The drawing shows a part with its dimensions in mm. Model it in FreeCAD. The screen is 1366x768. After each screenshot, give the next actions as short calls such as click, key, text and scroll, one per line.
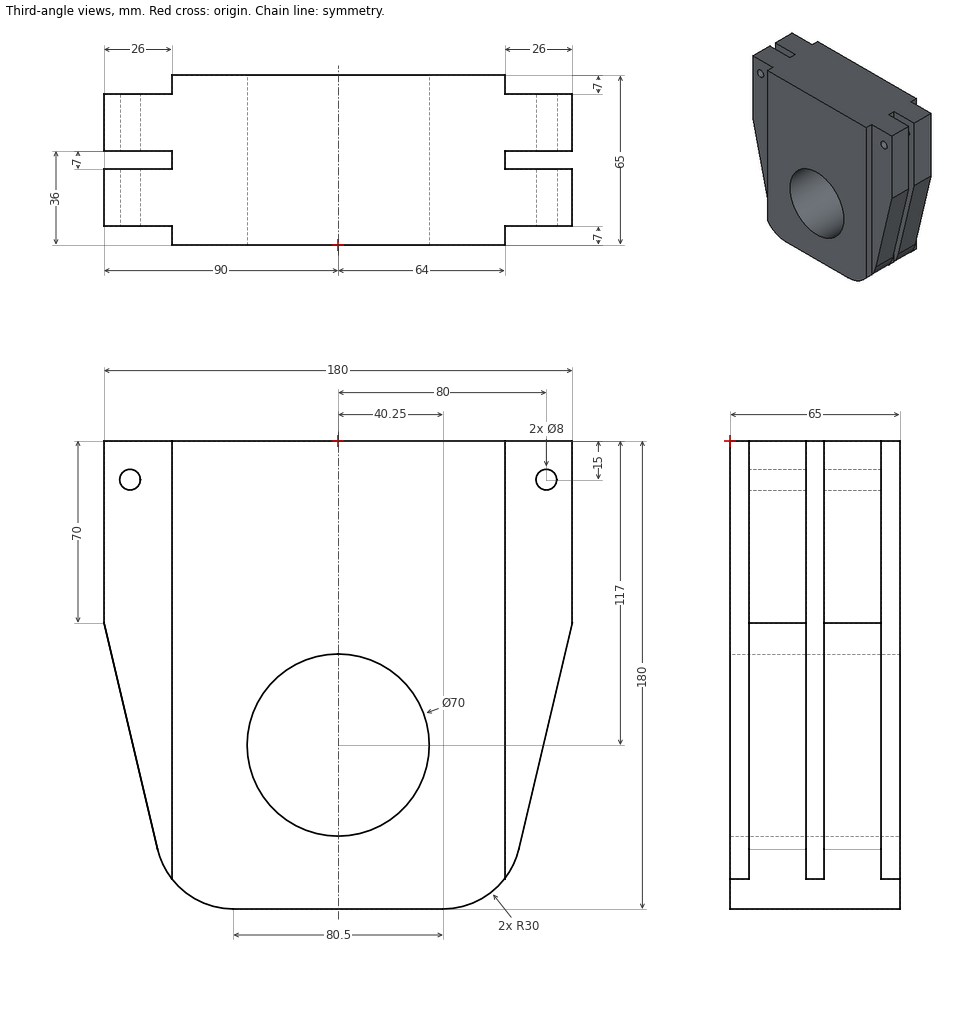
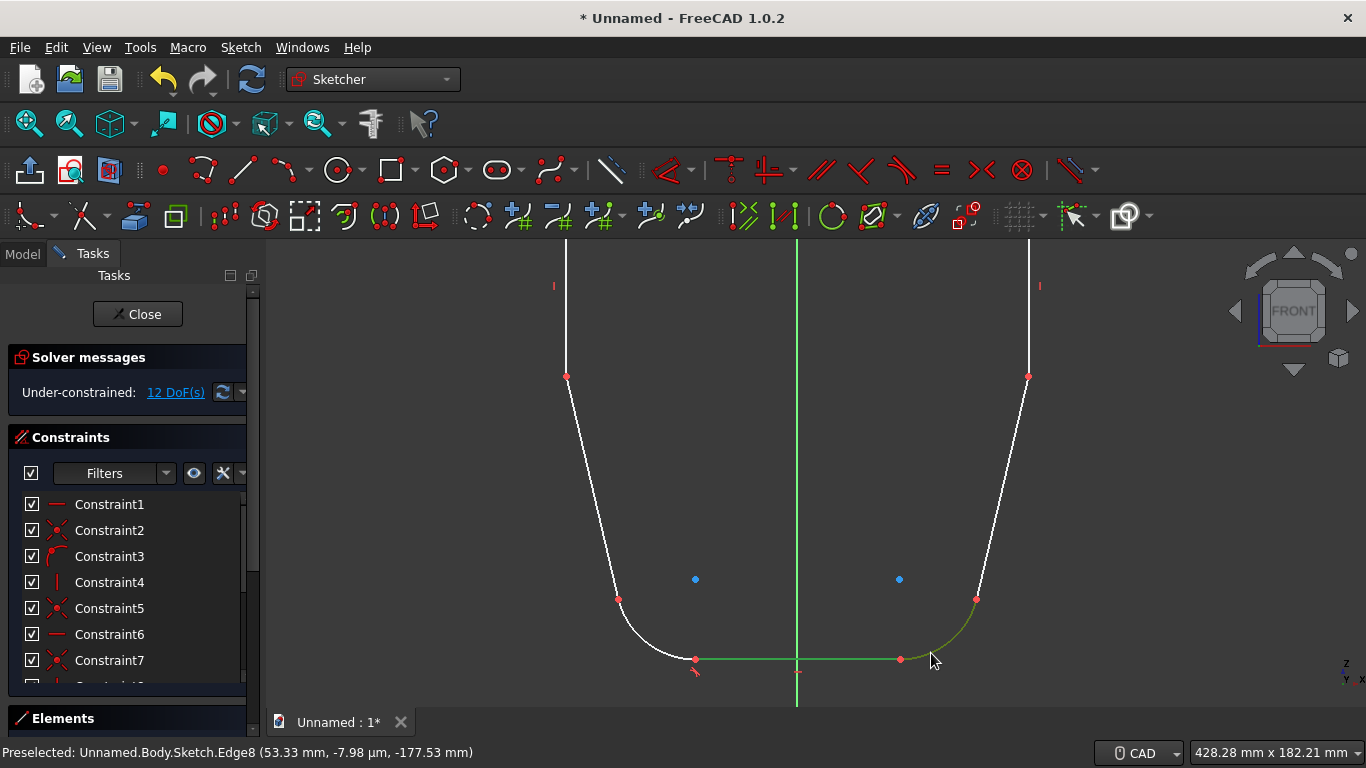
click(902, 170)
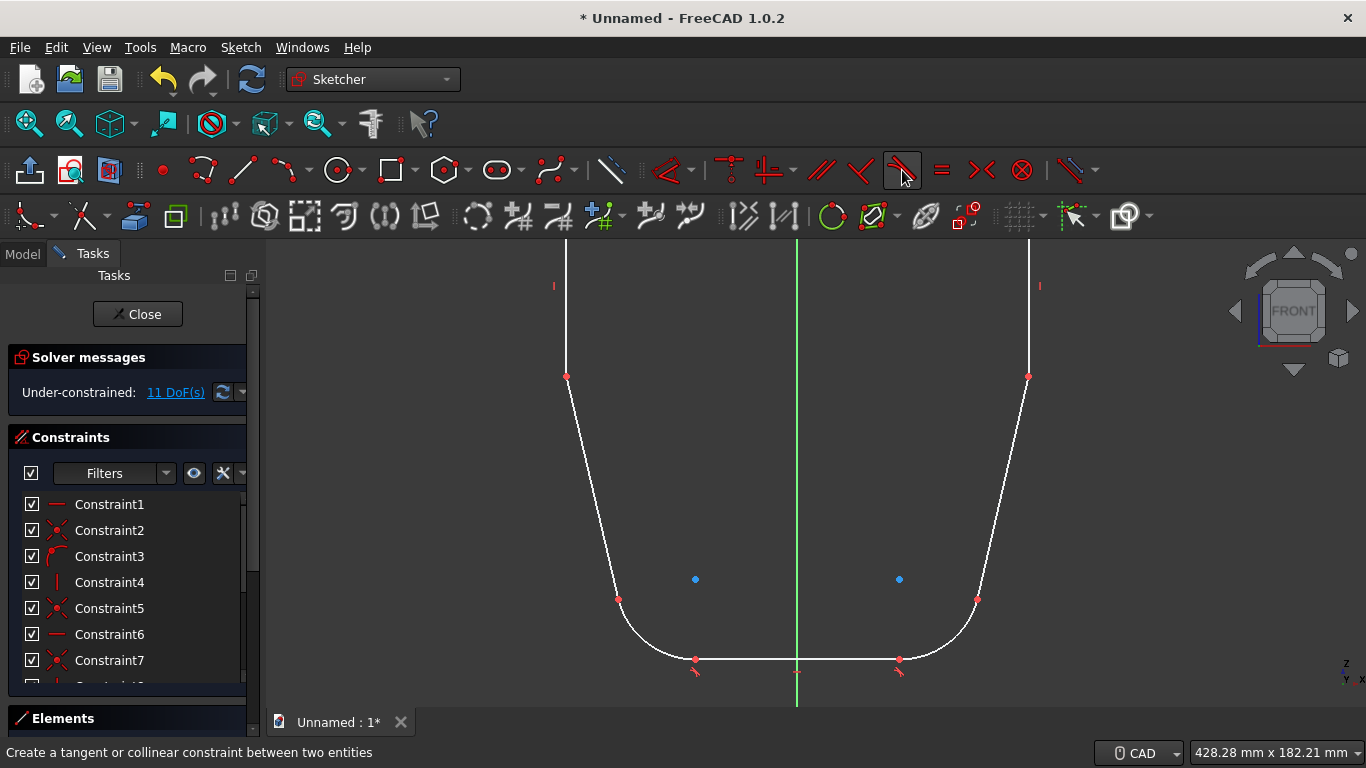
click(603, 533)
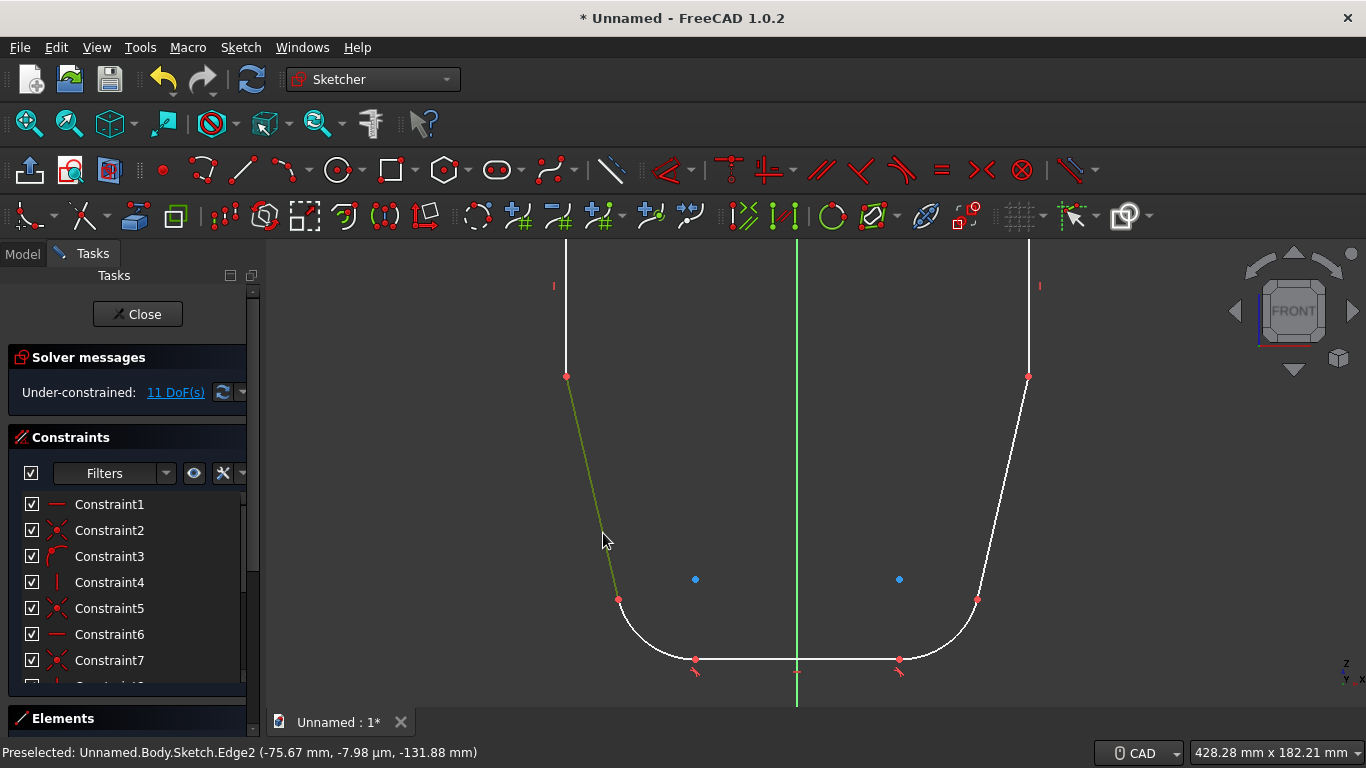
click(632, 628)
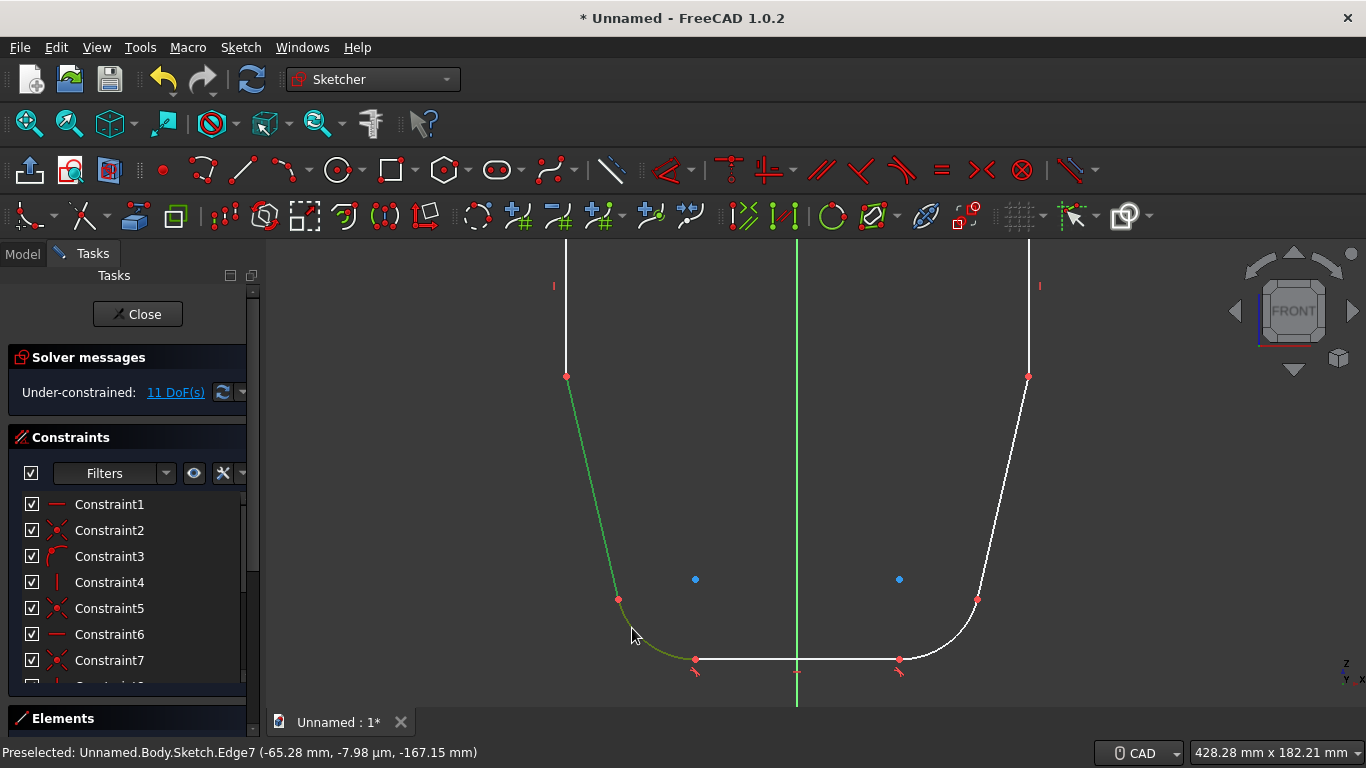
click(902, 170)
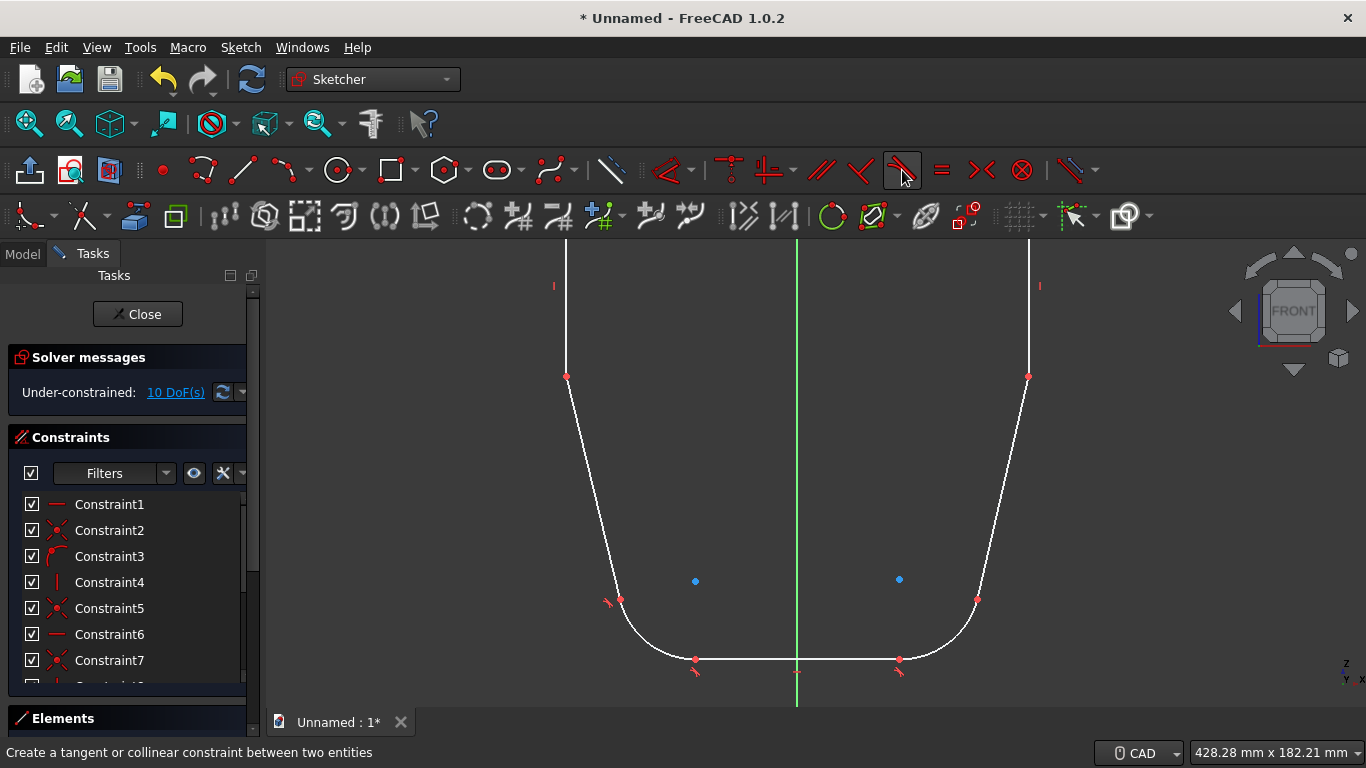
click(1013, 443)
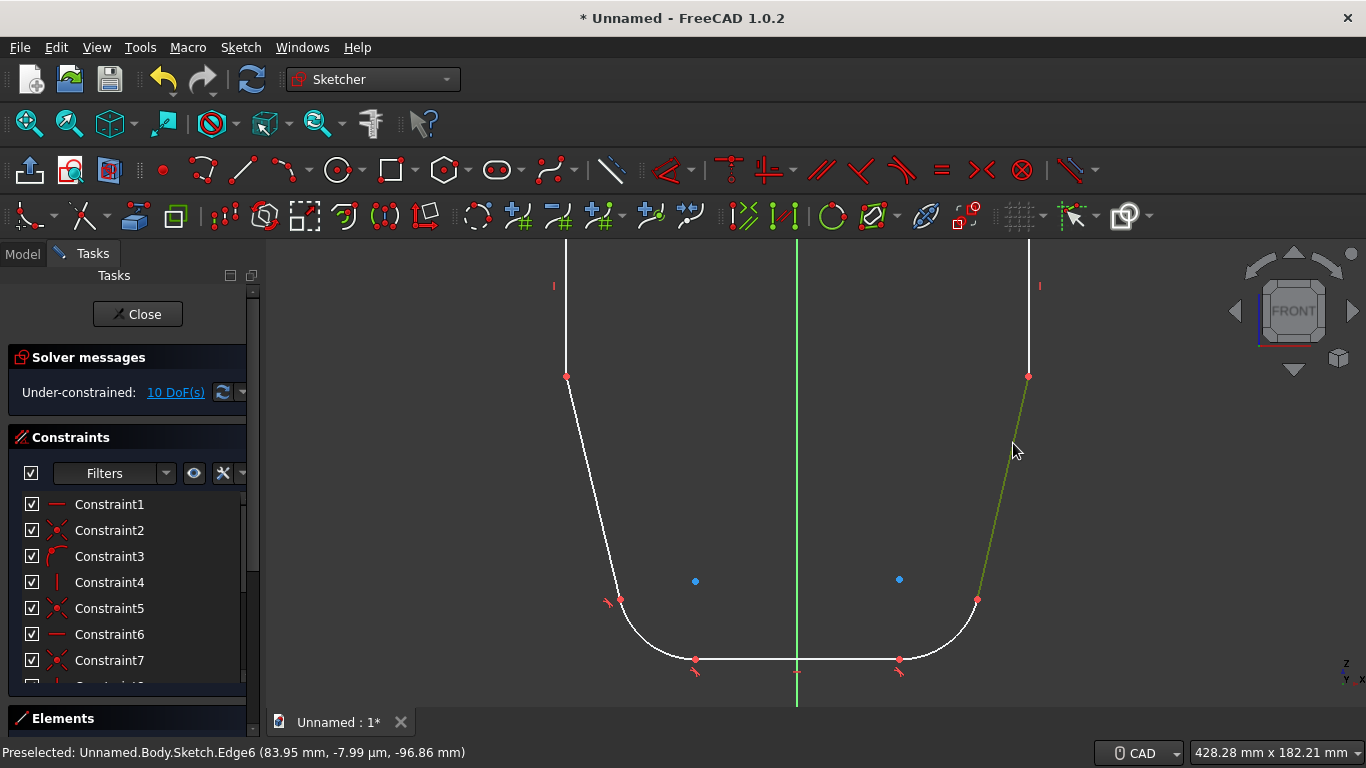
click(931, 653)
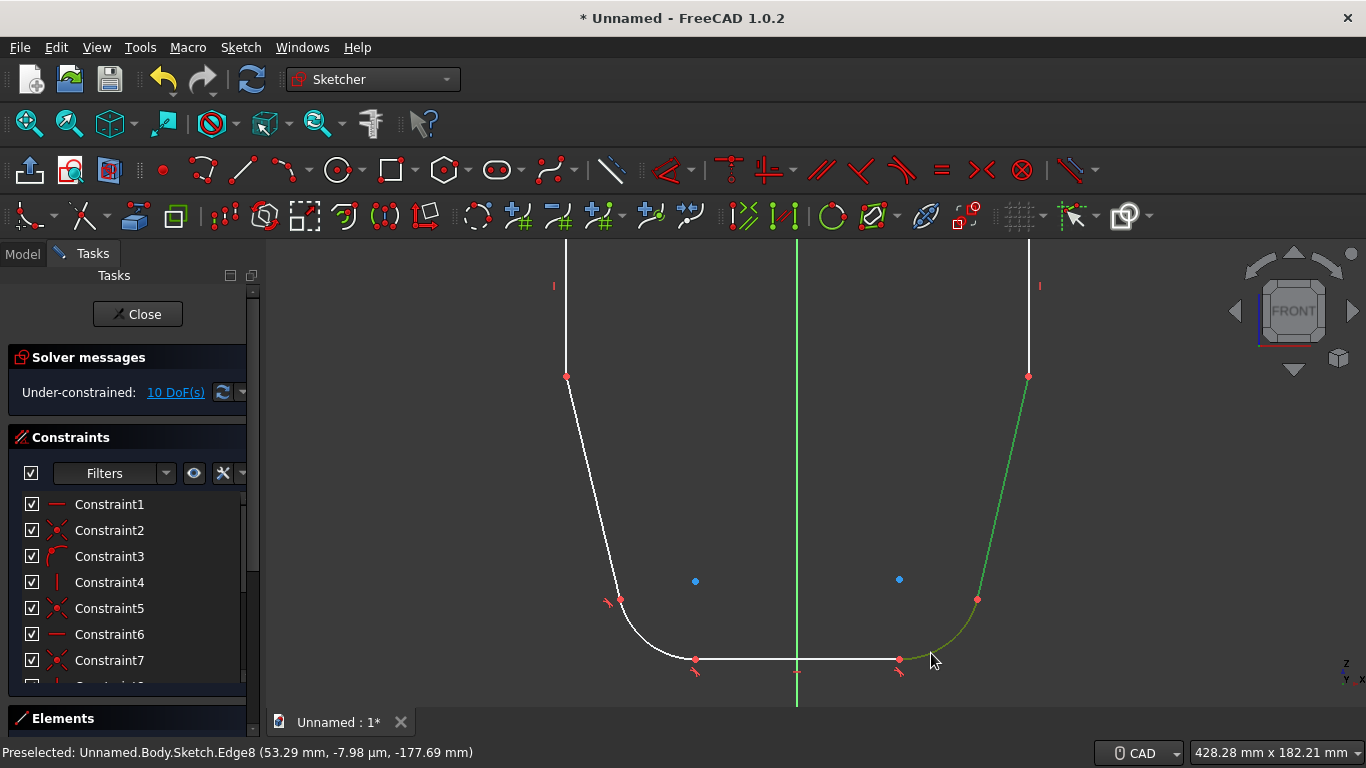
click(902, 170)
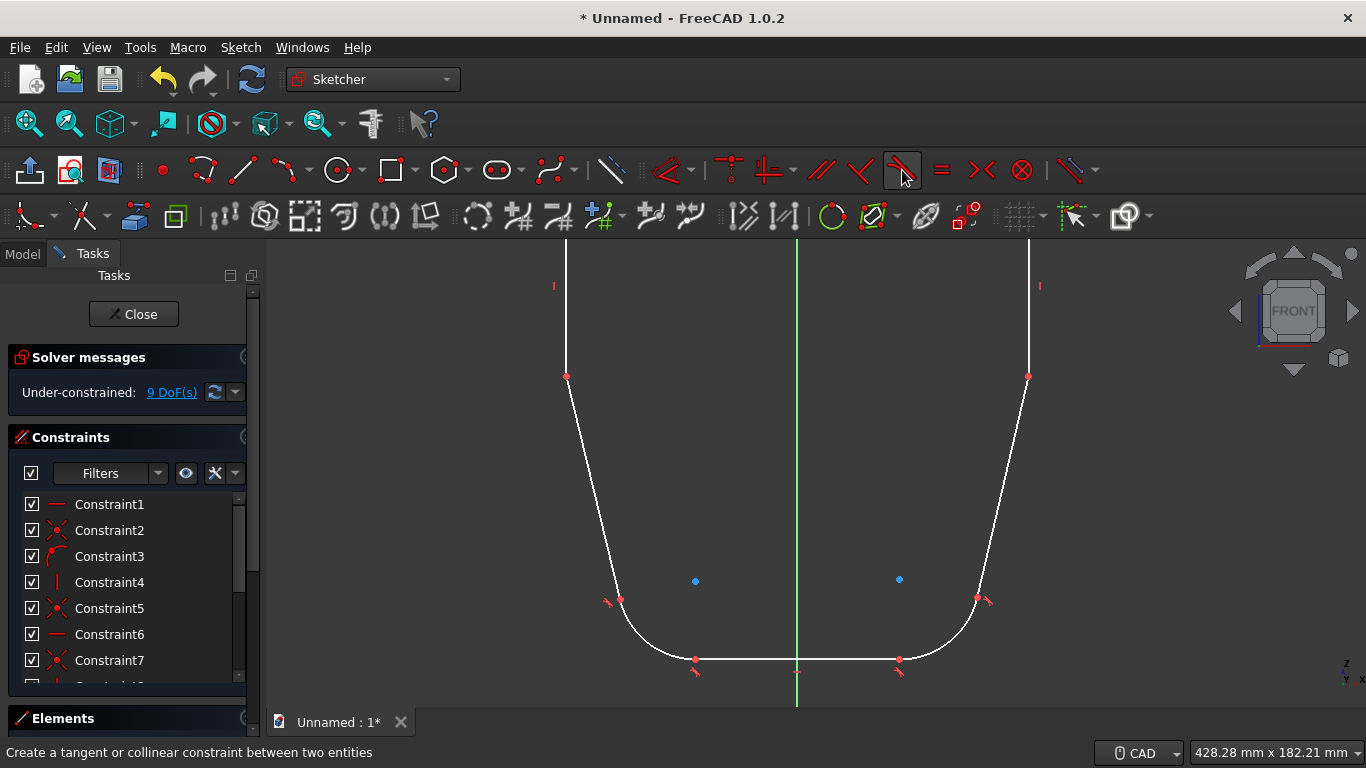
click(633, 628)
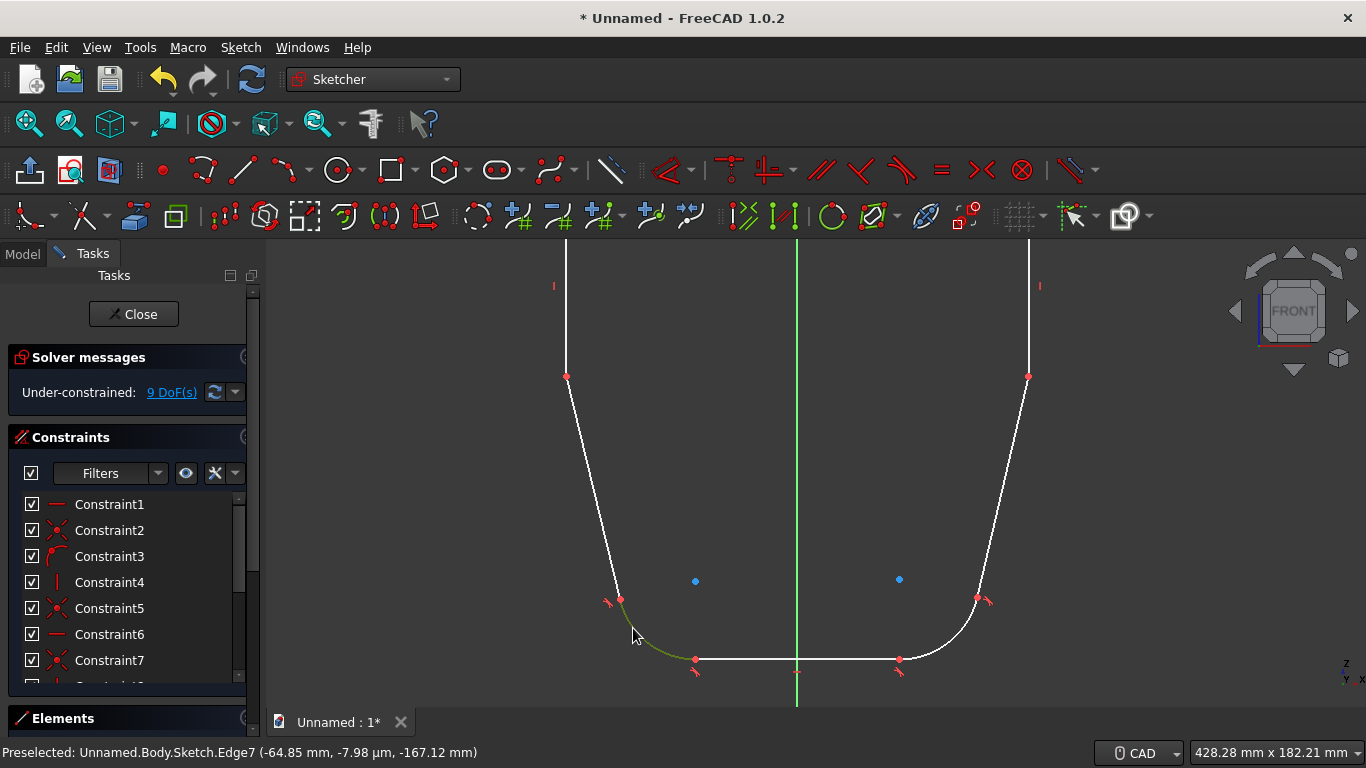
click(931, 653)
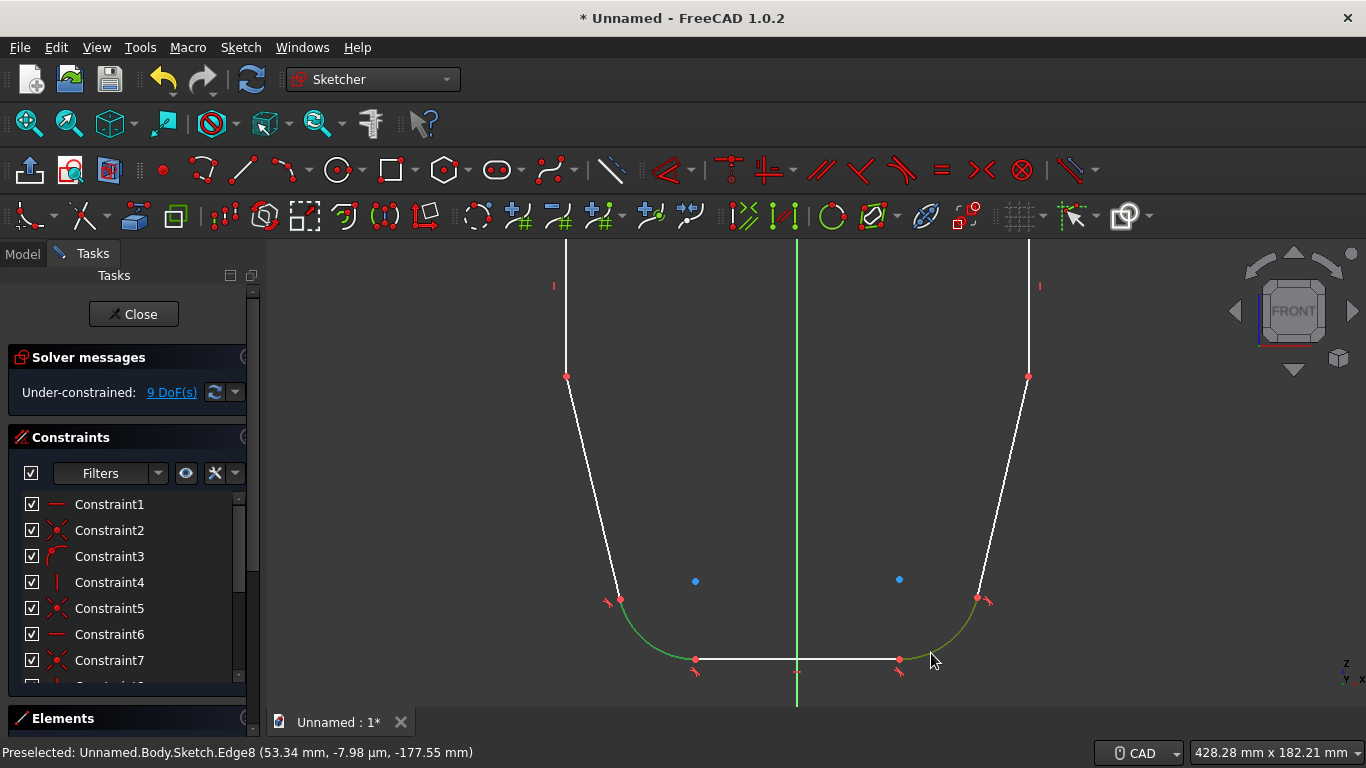
click(942, 170)